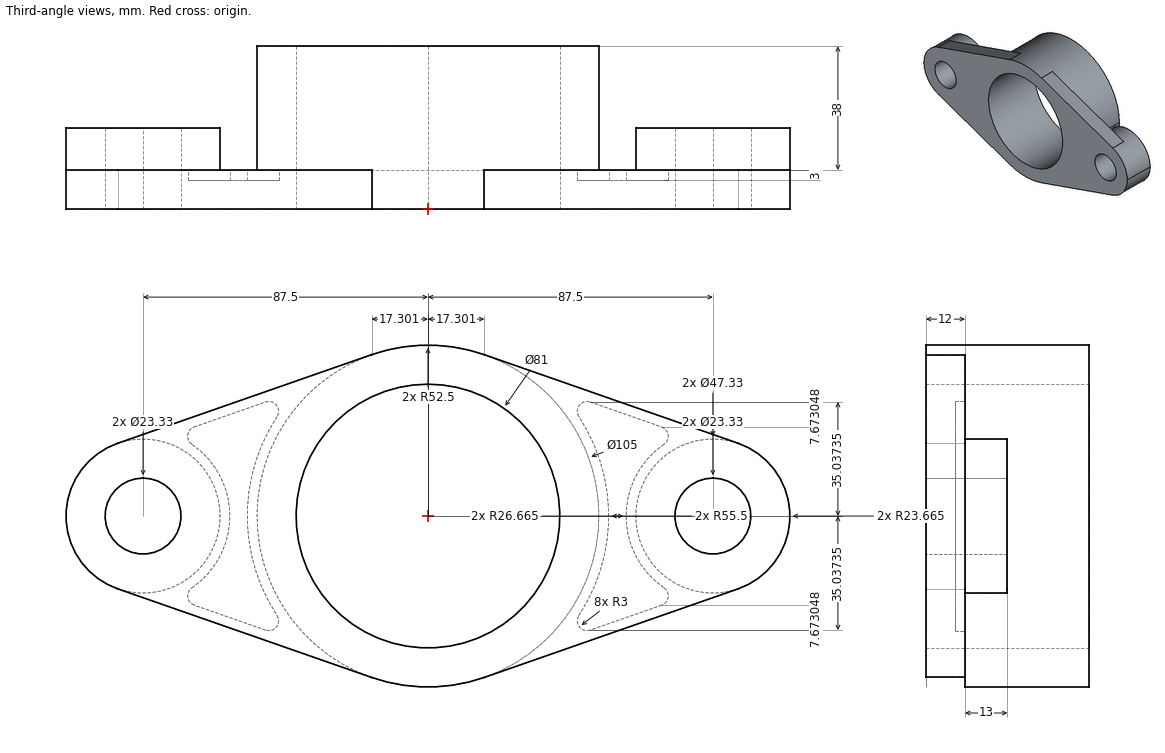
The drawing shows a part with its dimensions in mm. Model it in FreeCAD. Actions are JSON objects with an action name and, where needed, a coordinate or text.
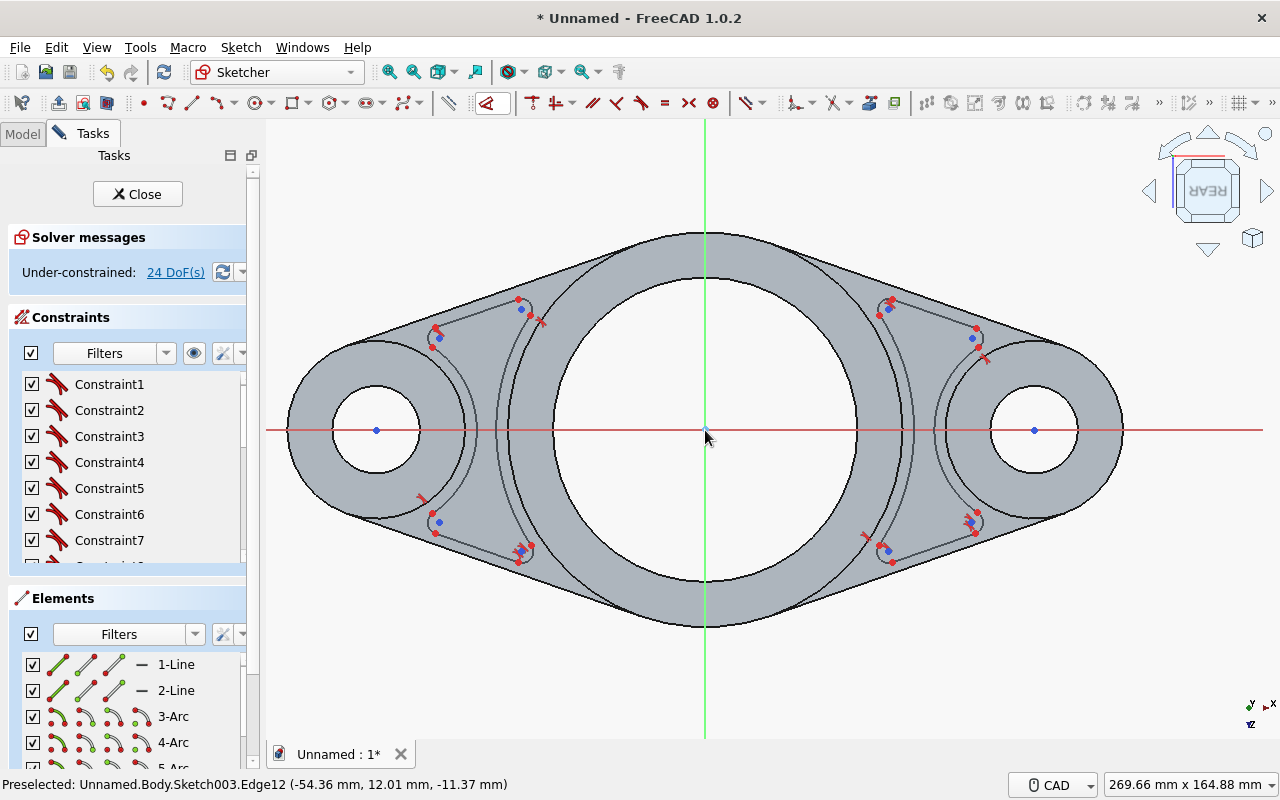
{"action": "scroll", "coordinate": [884, 300], "scroll_direction": "up", "scroll_amount": 3}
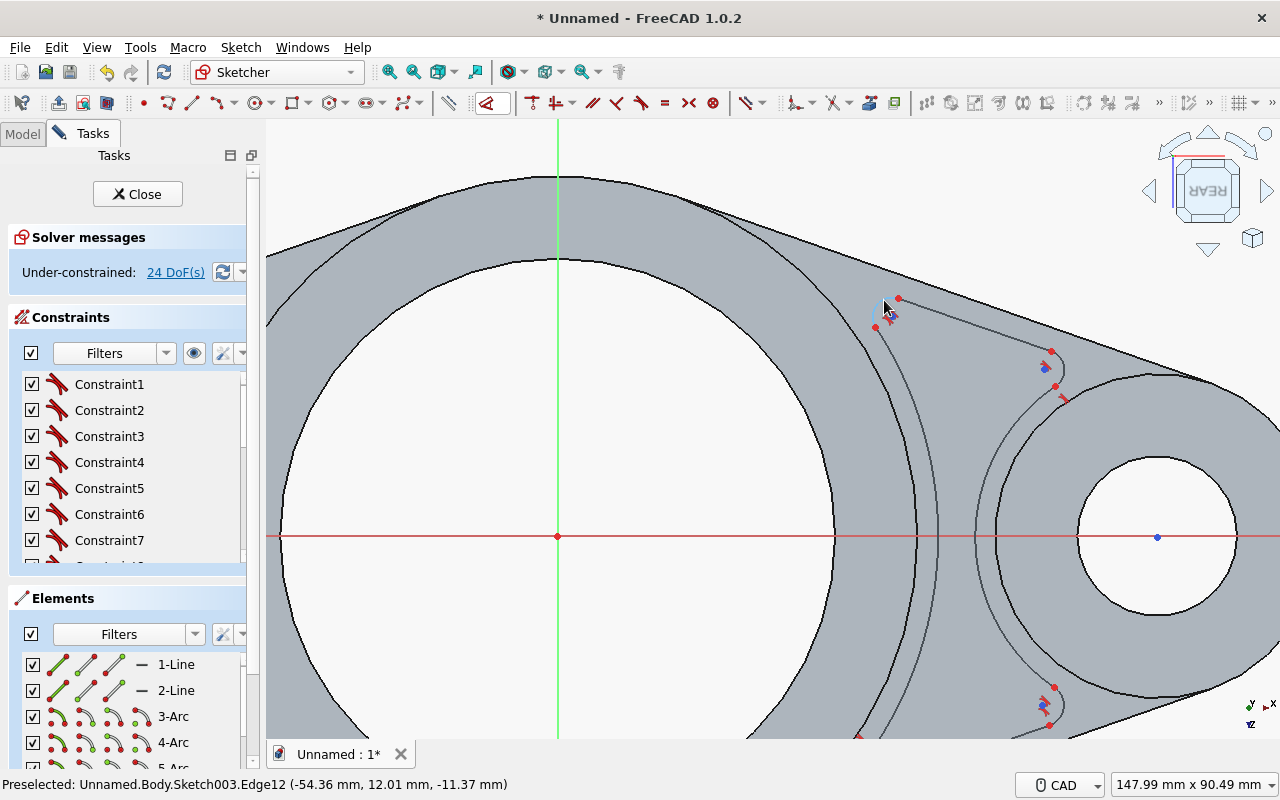
{"action": "left_click", "coordinate": [884, 299]}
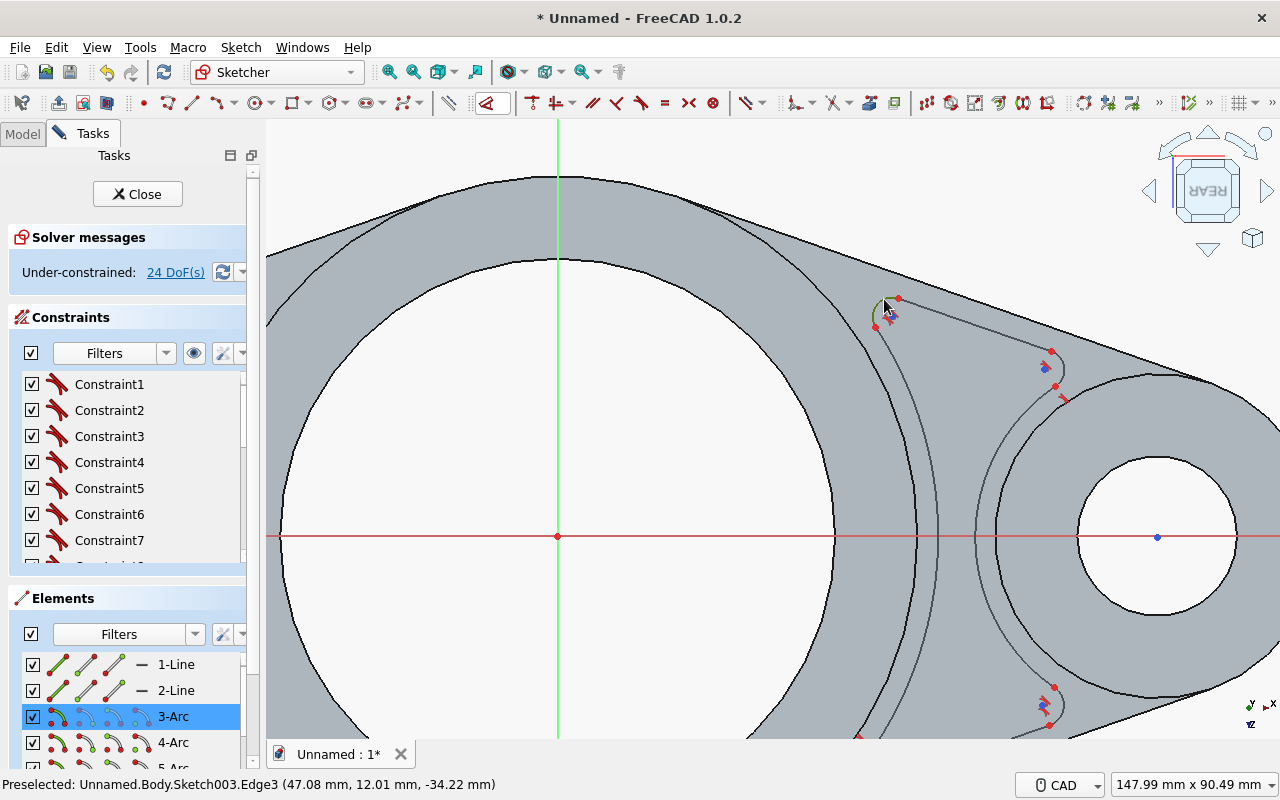
{"action": "scroll", "coordinate": [883, 299], "scroll_direction": "down", "scroll_amount": 3}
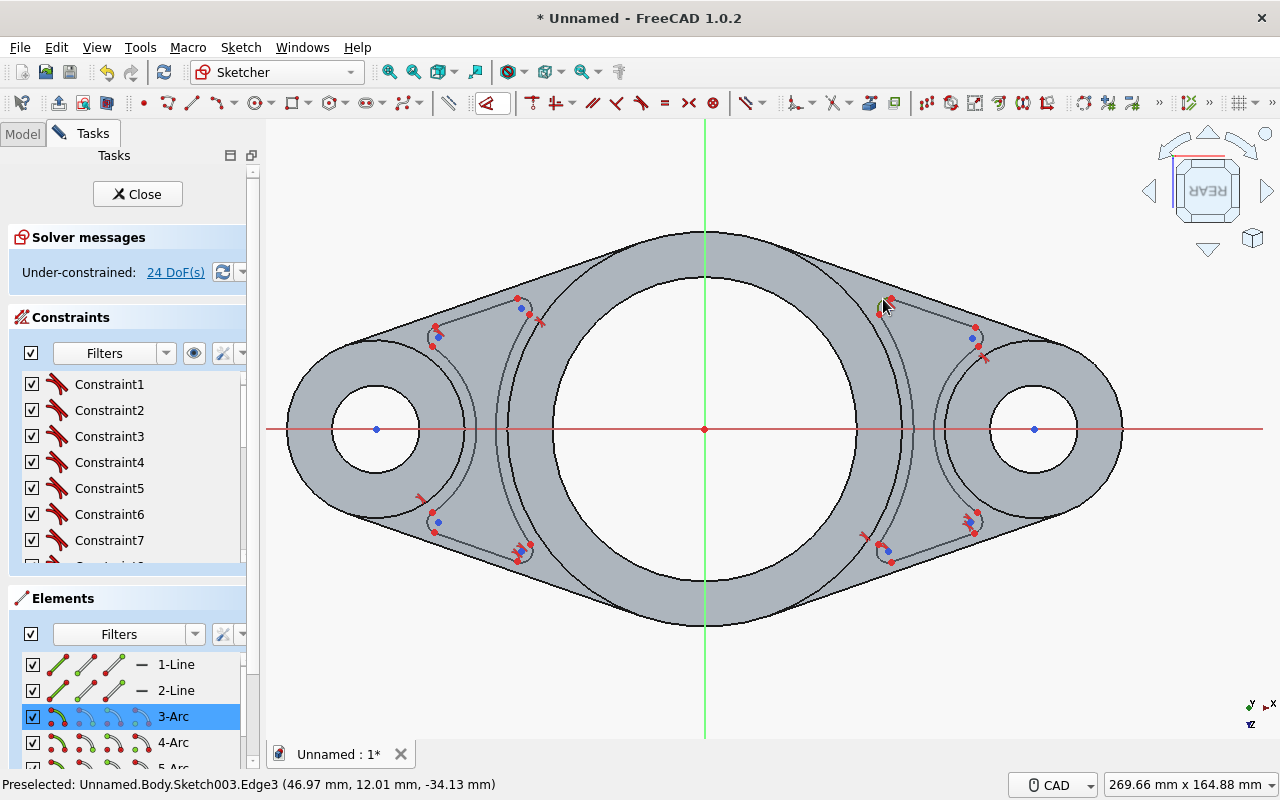
{"action": "scroll", "coordinate": [877, 553], "scroll_direction": "up", "scroll_amount": 3}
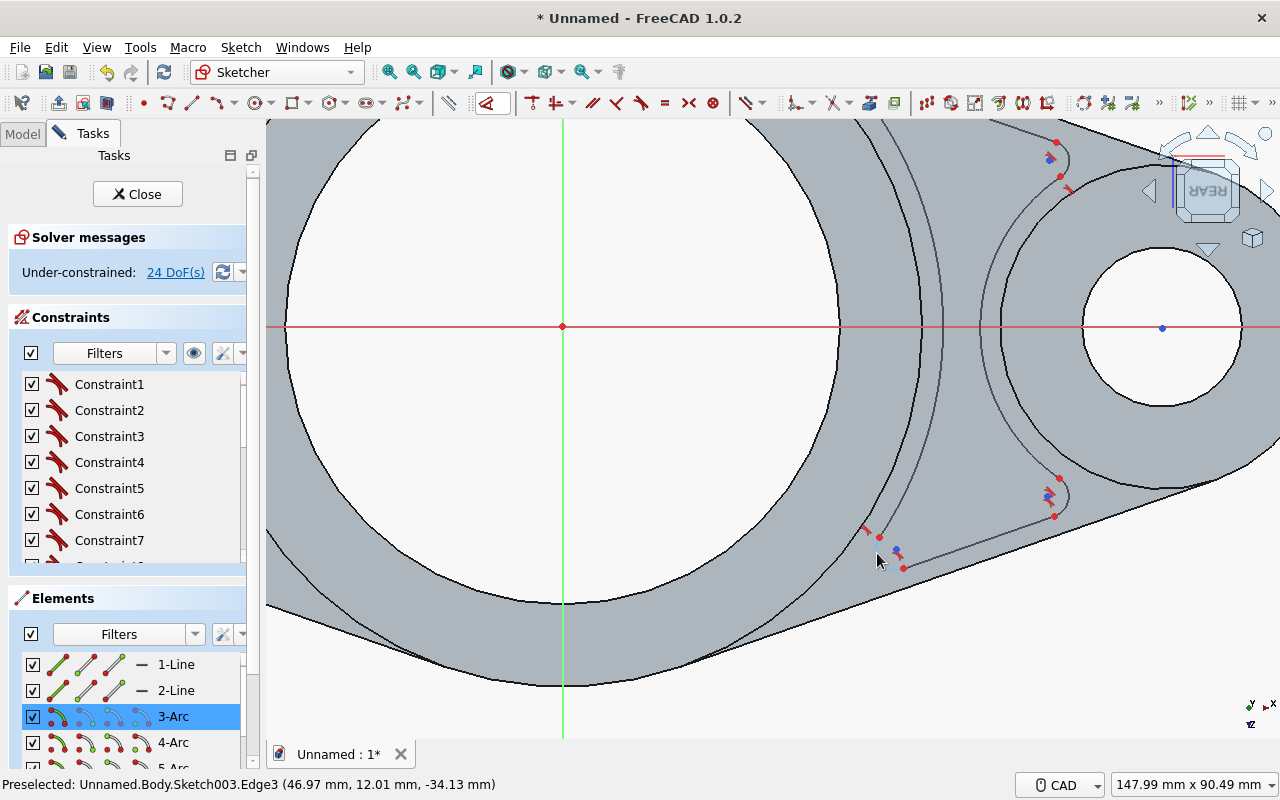
{"action": "left_click", "coordinate": [876, 553]}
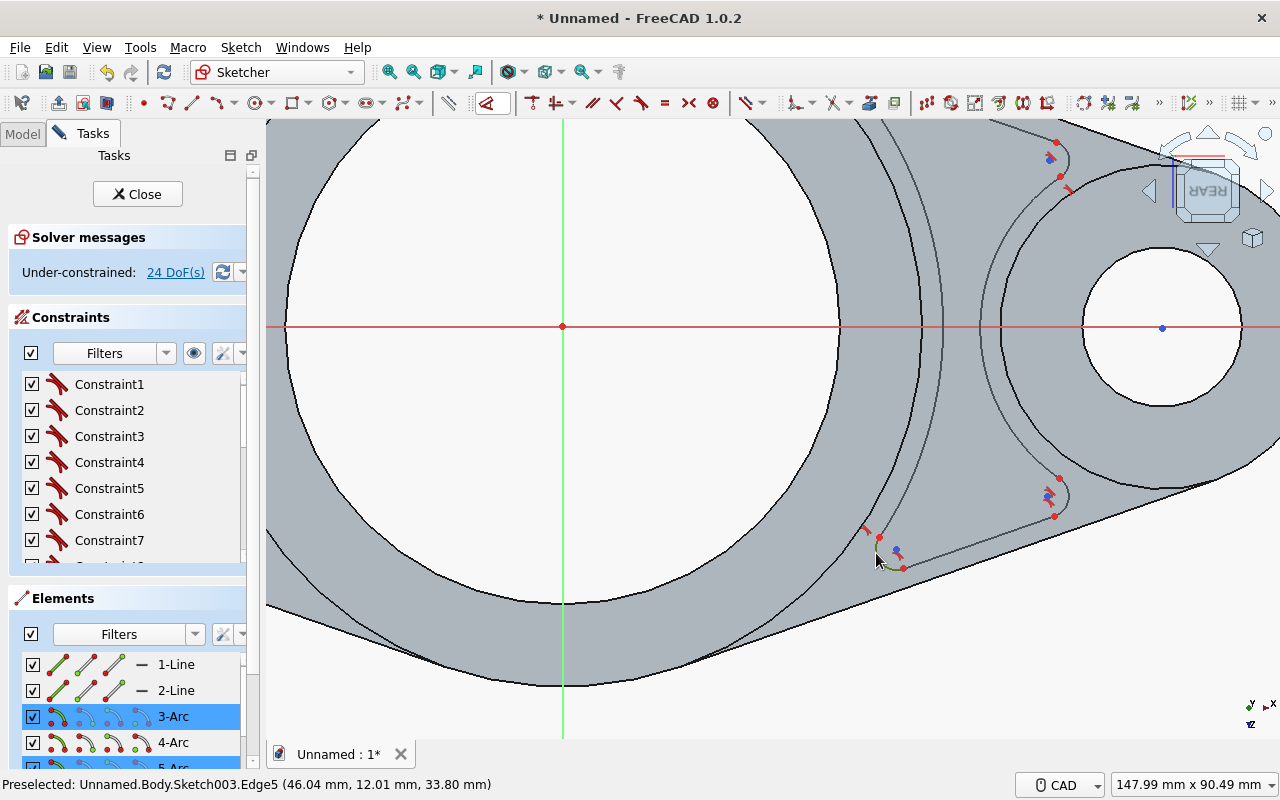
{"action": "left_click", "coordinate": [1065, 508]}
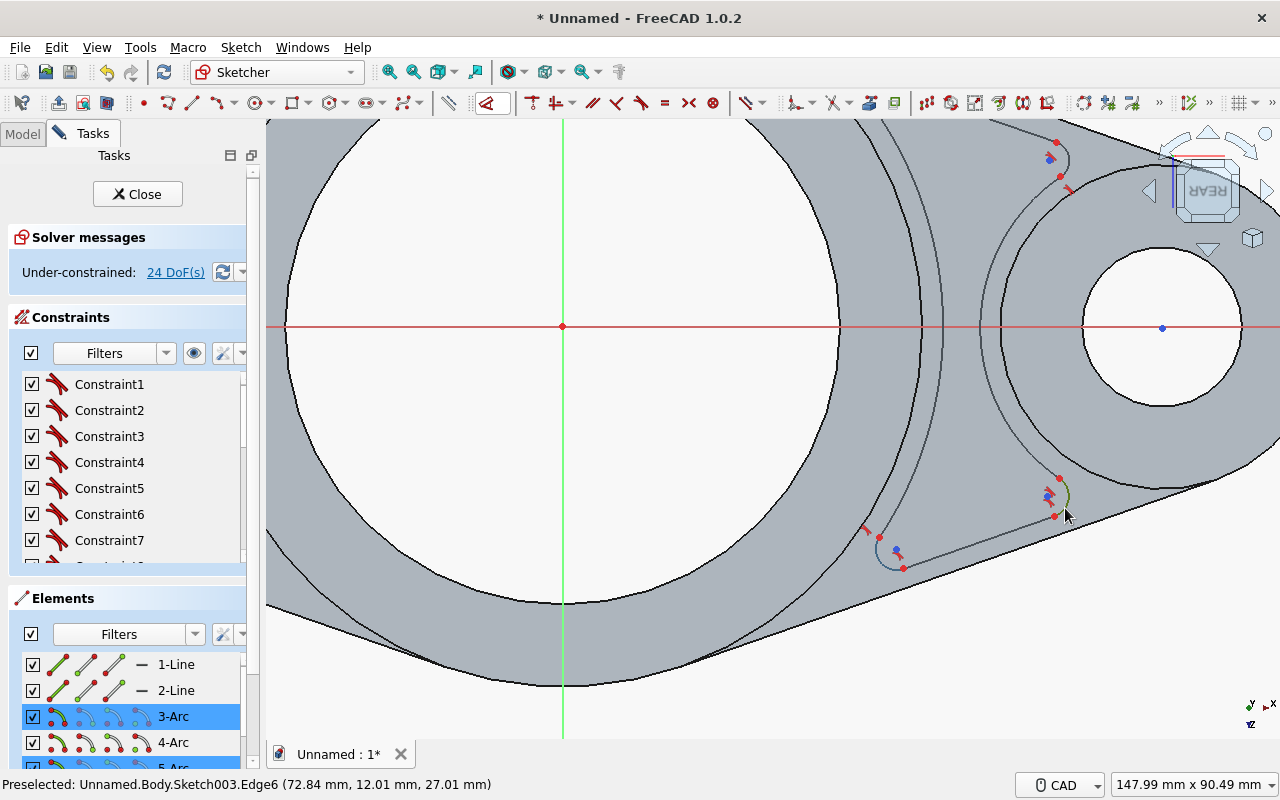
{"action": "left_click", "coordinate": [1068, 167]}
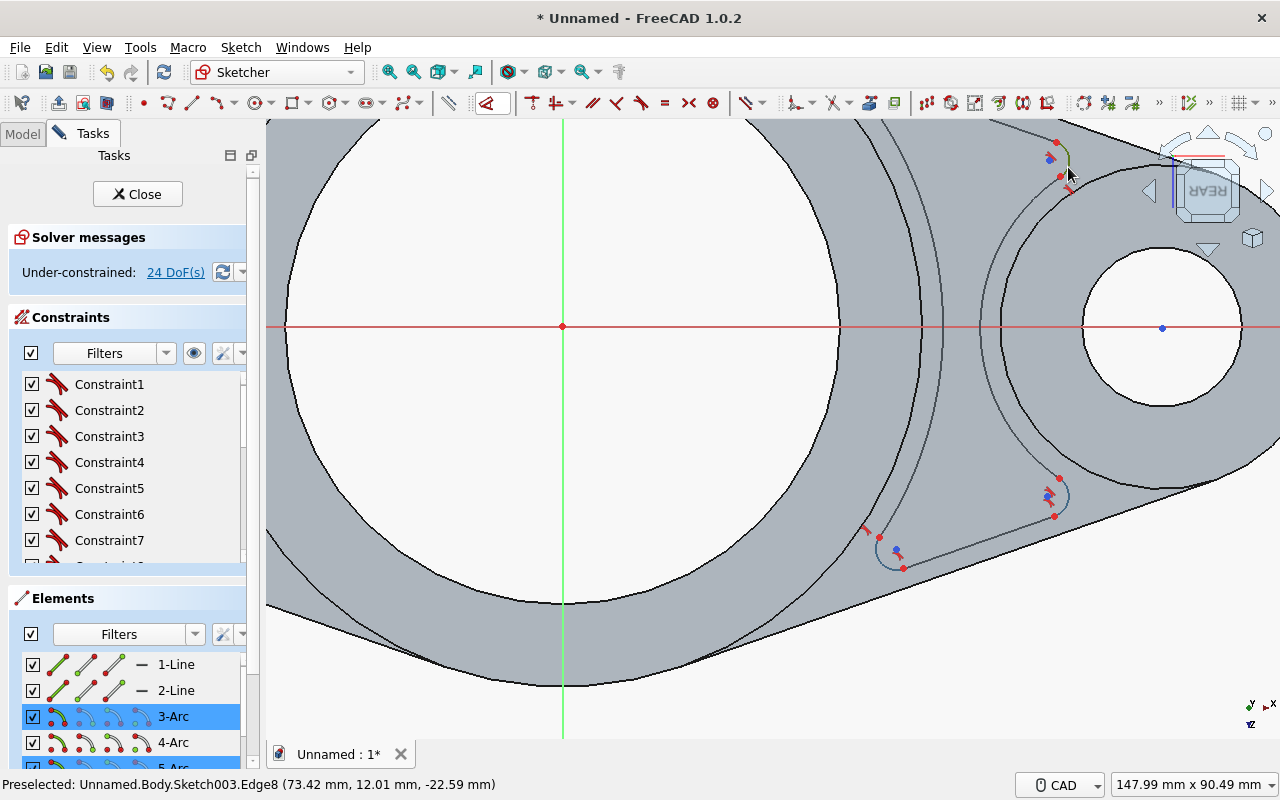
{"action": "scroll", "coordinate": [877, 553], "scroll_direction": "down", "scroll_amount": 3}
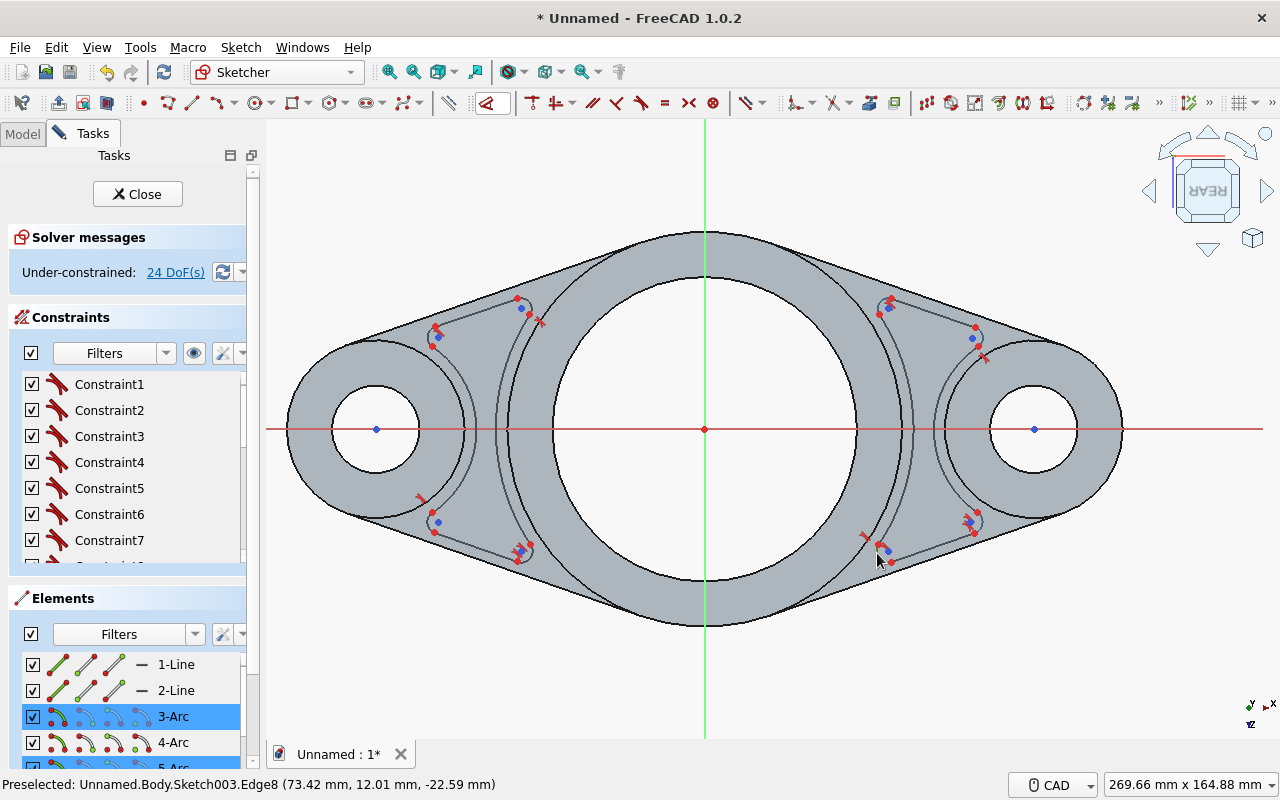
{"action": "scroll", "coordinate": [526, 562], "scroll_direction": "up", "scroll_amount": 3}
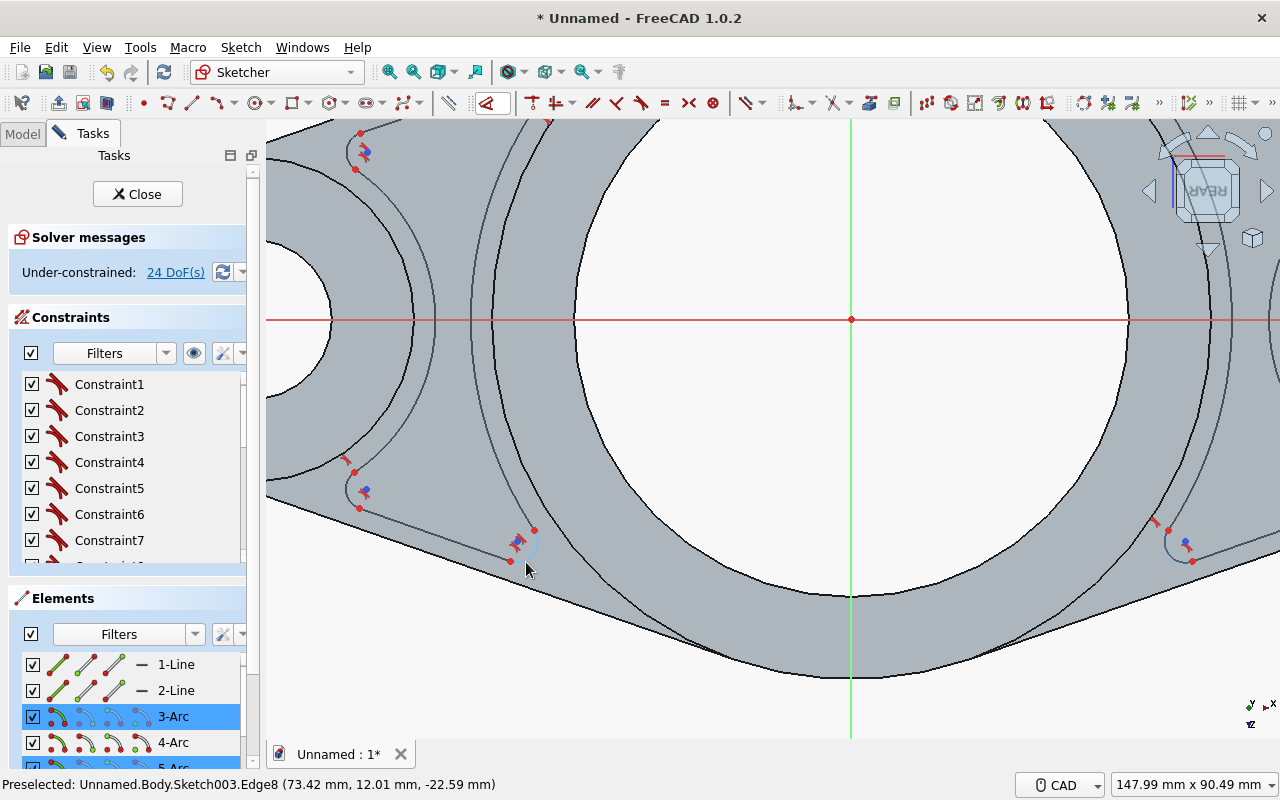
{"action": "left_click", "coordinate": [526, 561]}